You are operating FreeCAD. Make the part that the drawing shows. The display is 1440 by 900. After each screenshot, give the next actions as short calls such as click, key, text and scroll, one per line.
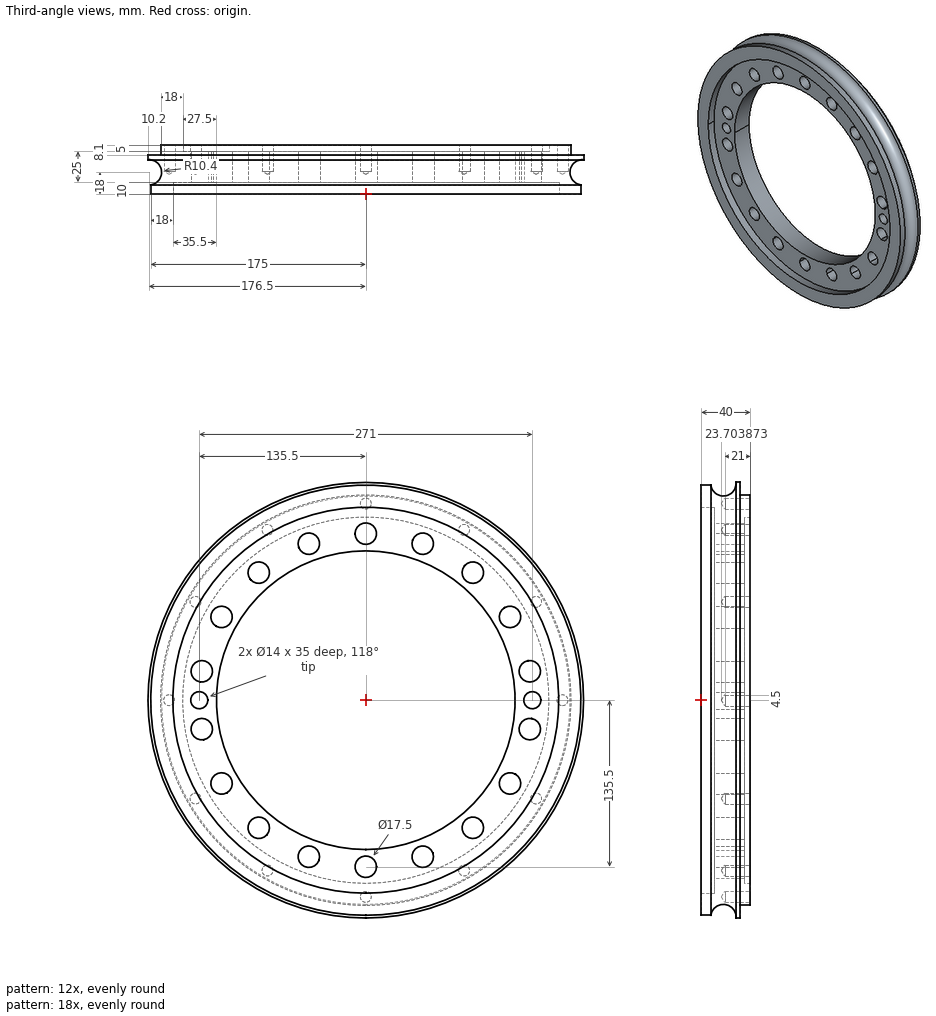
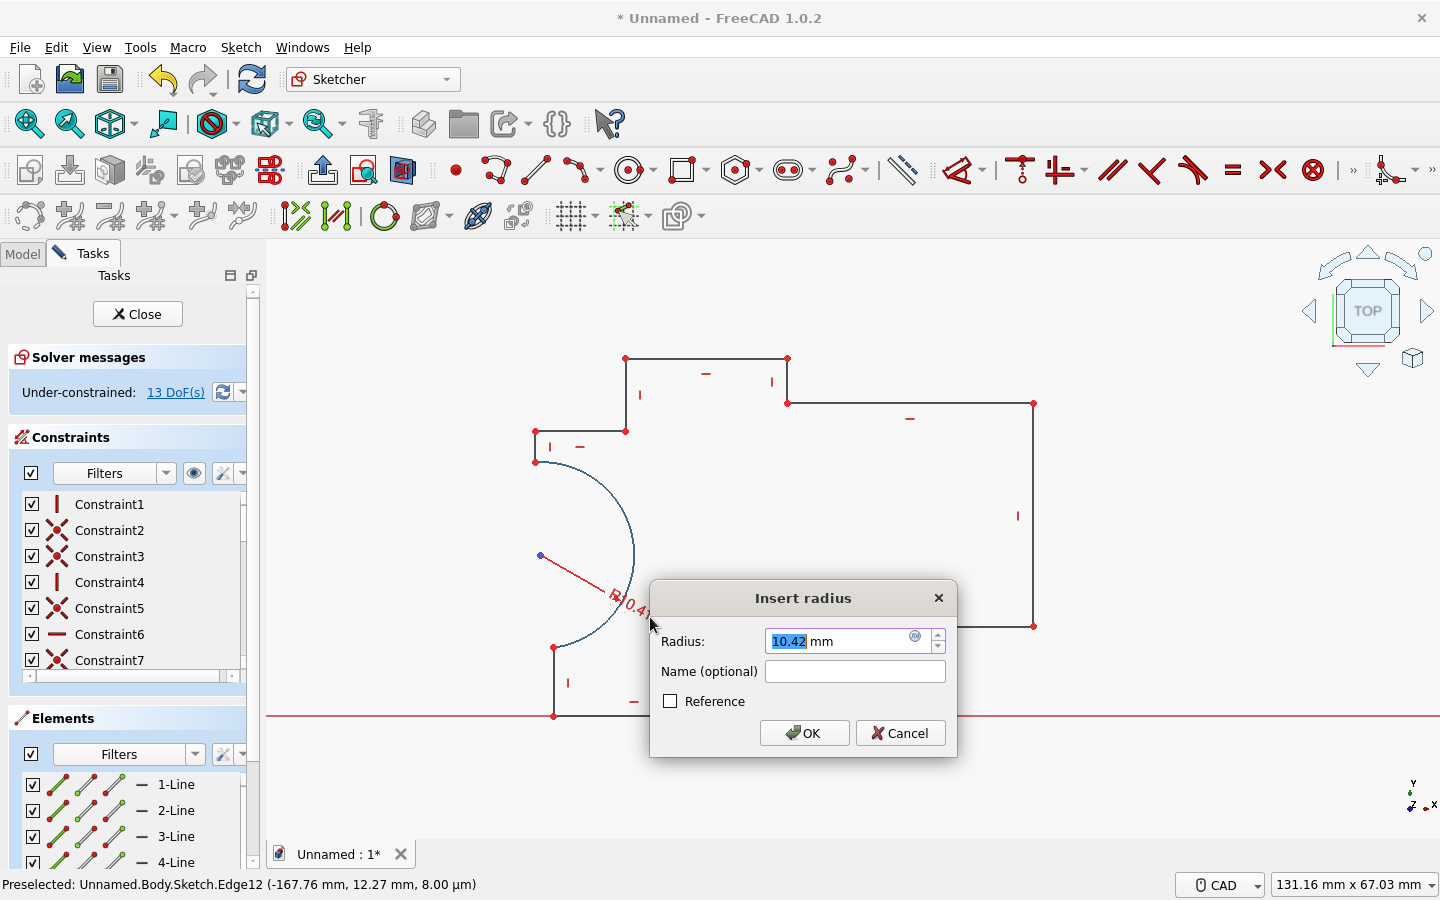
text(10.4)
key(Return)
key(Escape)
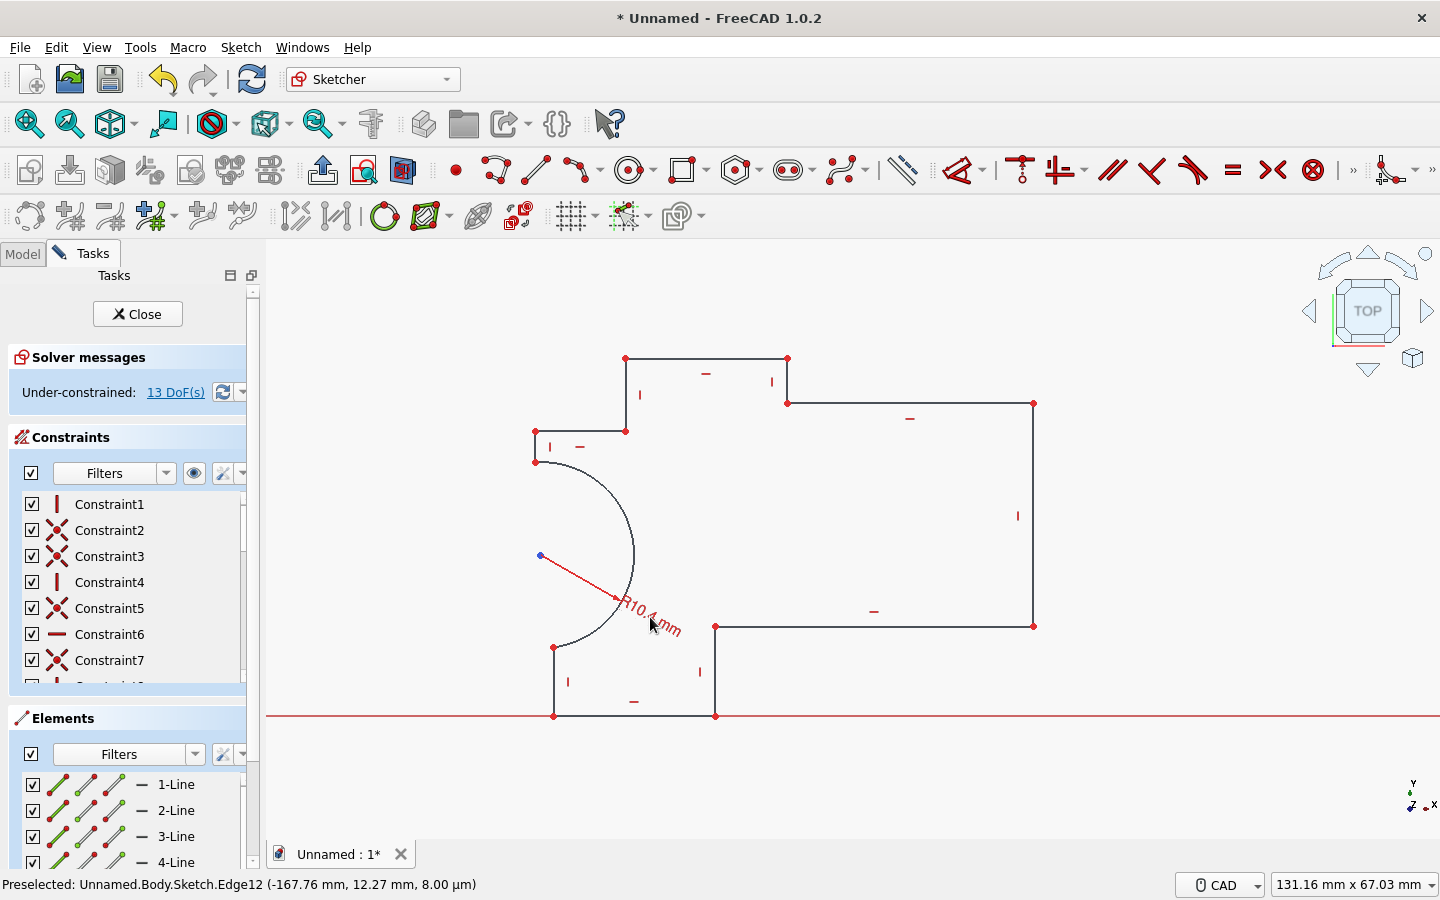
click(554, 716)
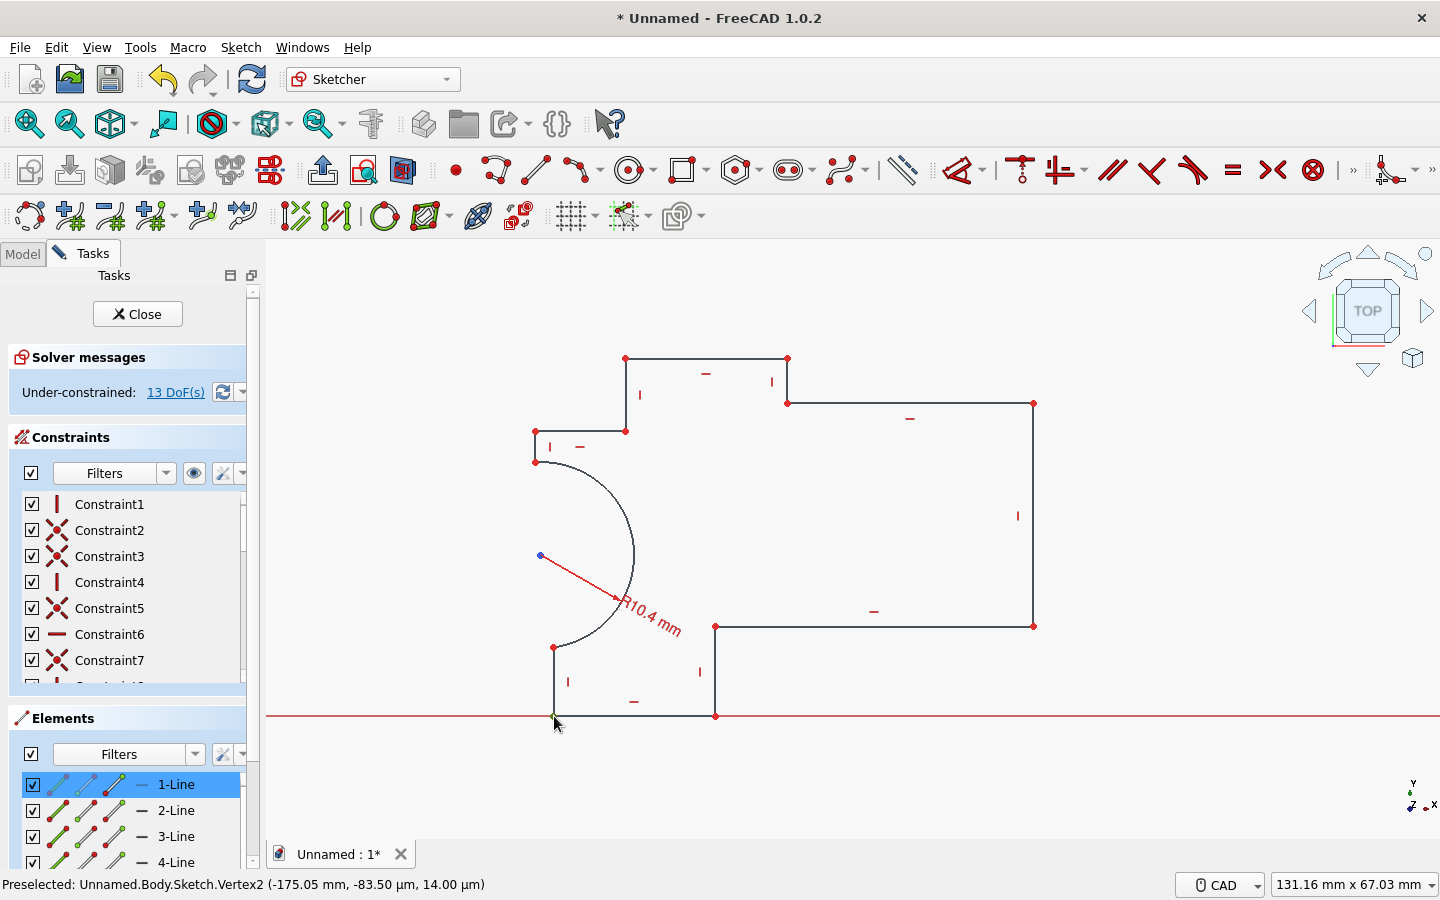
click(364, 716)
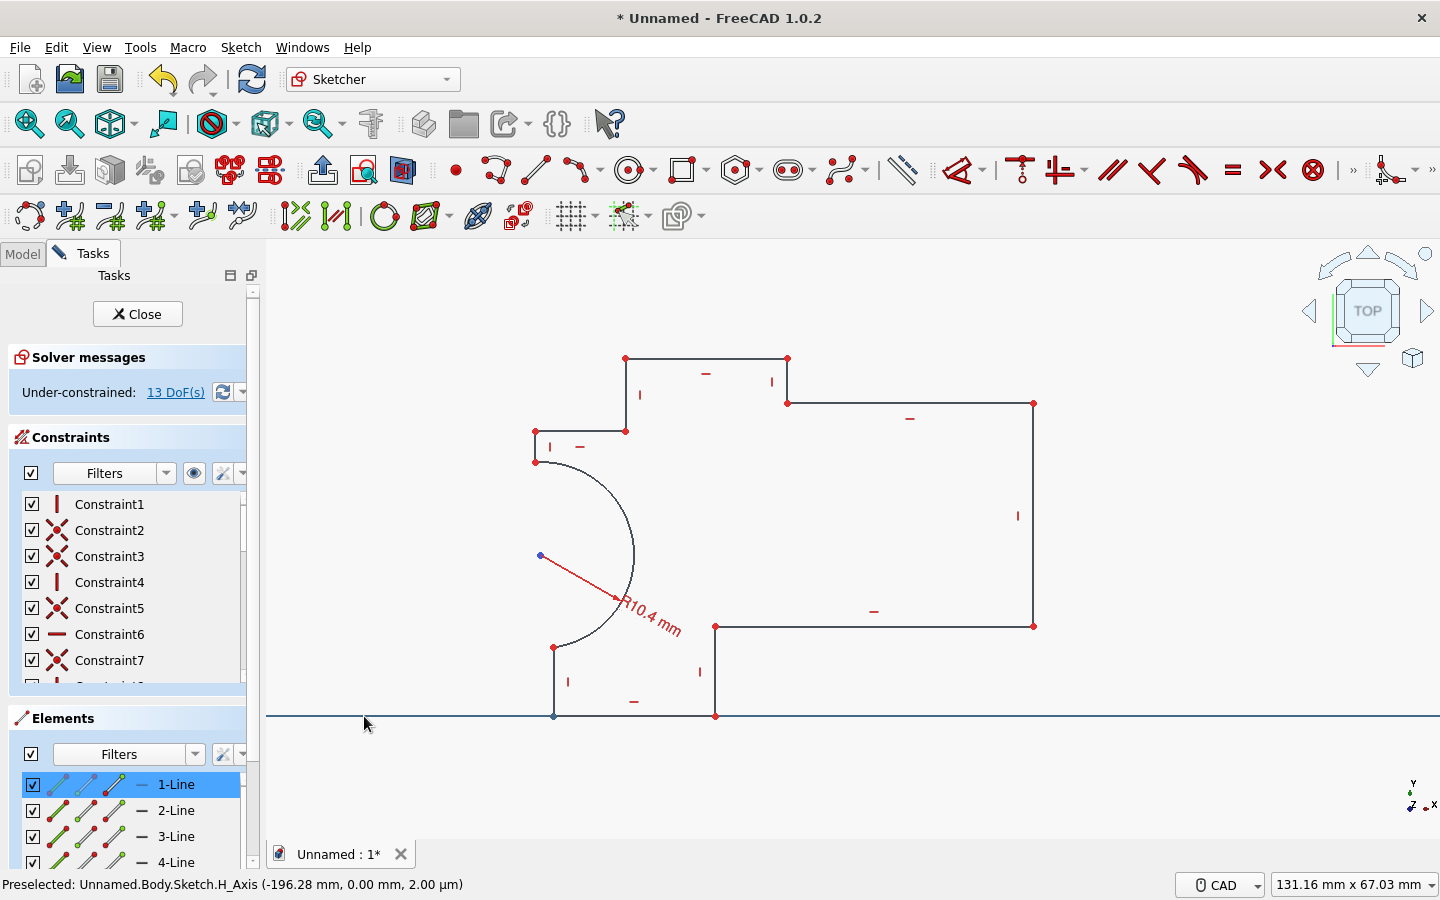
click(1020, 170)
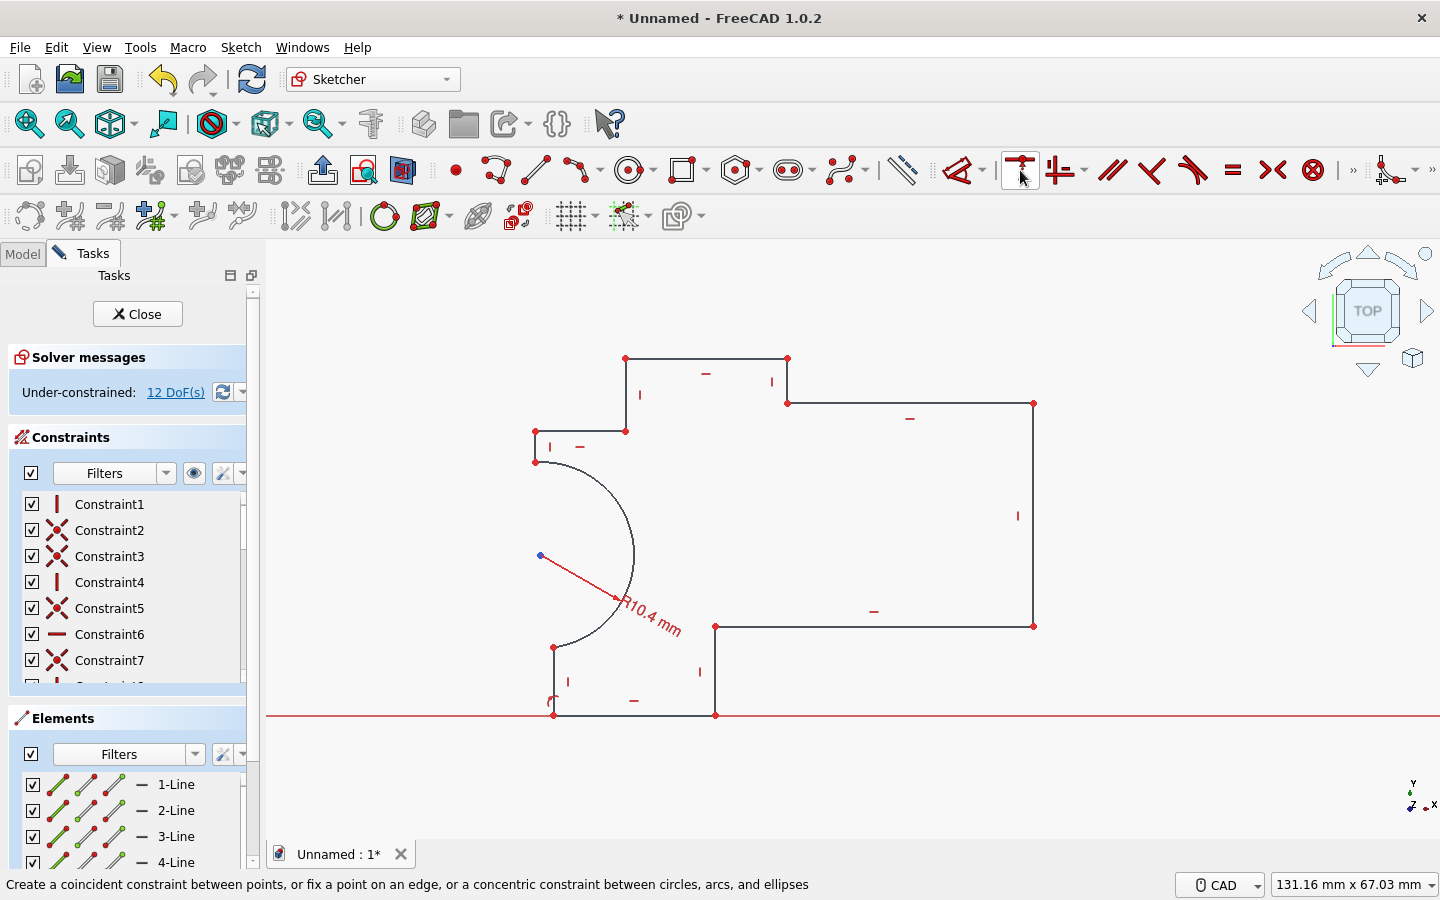
click(958, 170)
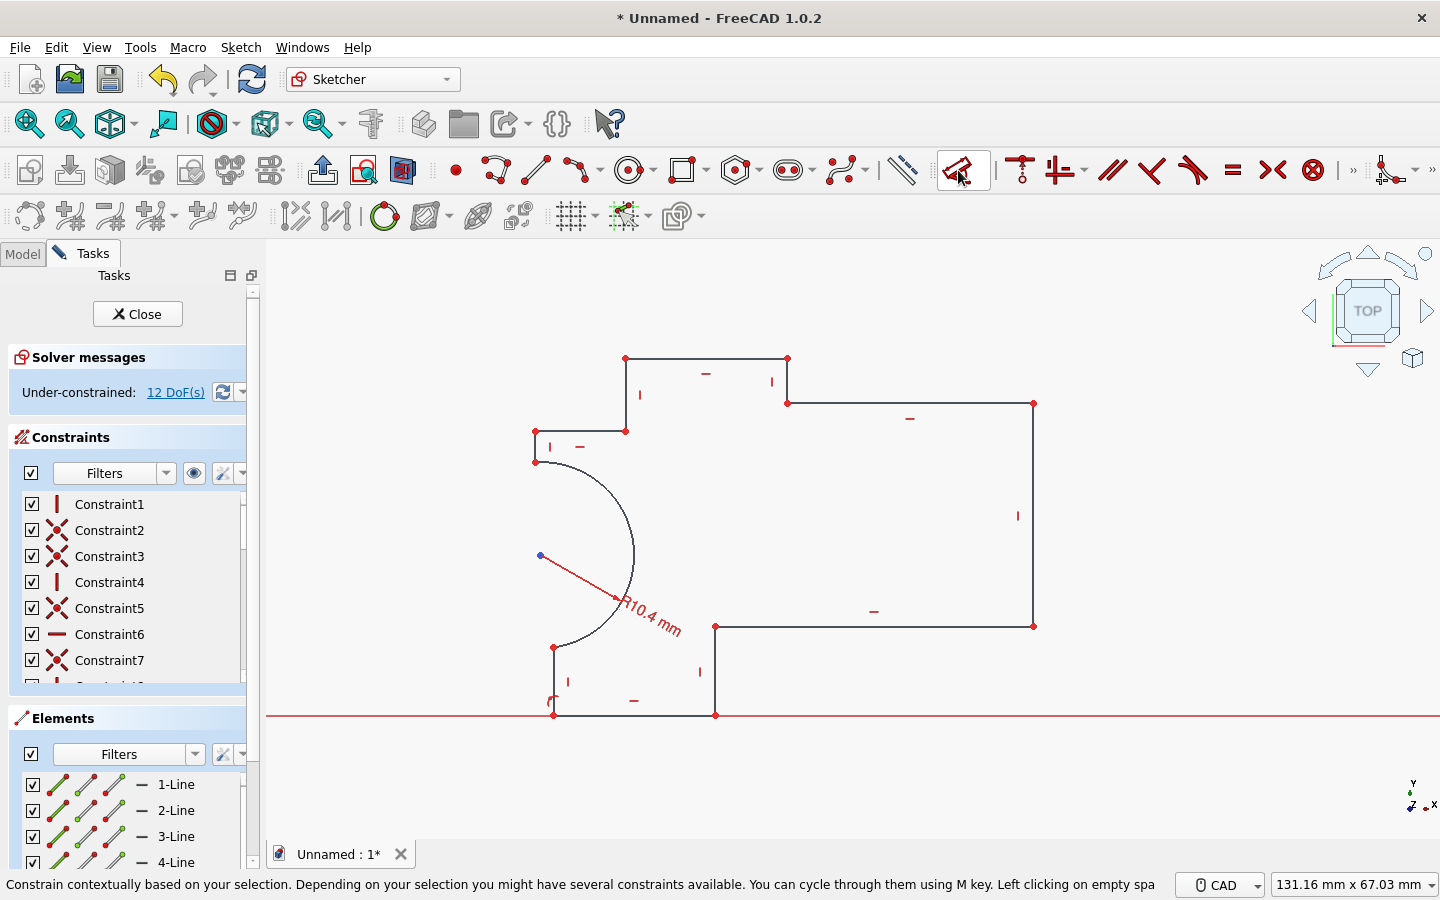
click(787, 390)
click(821, 381)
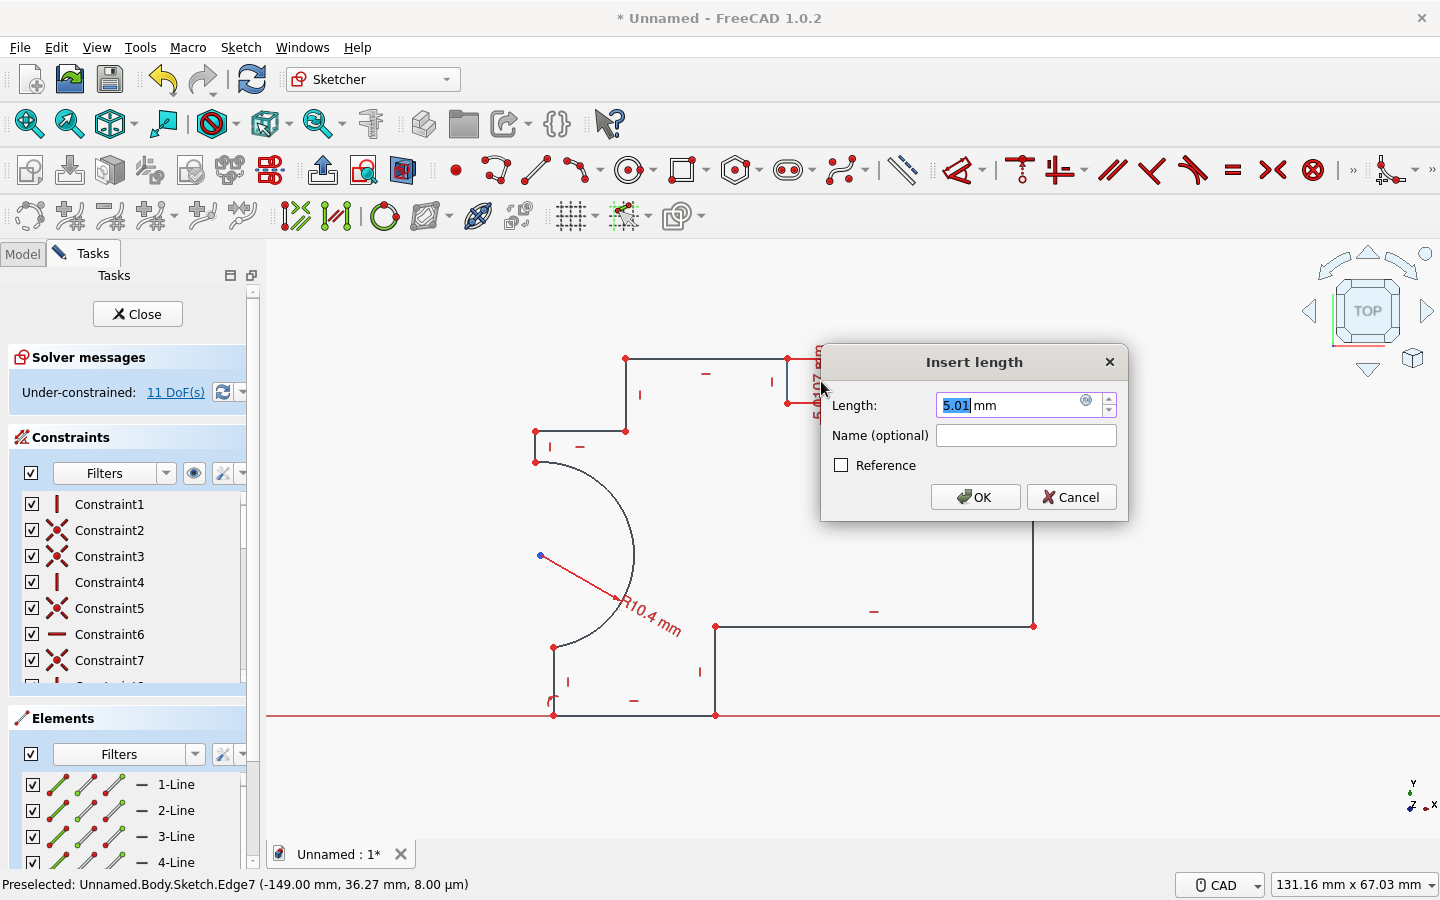
text(5)
key(Return)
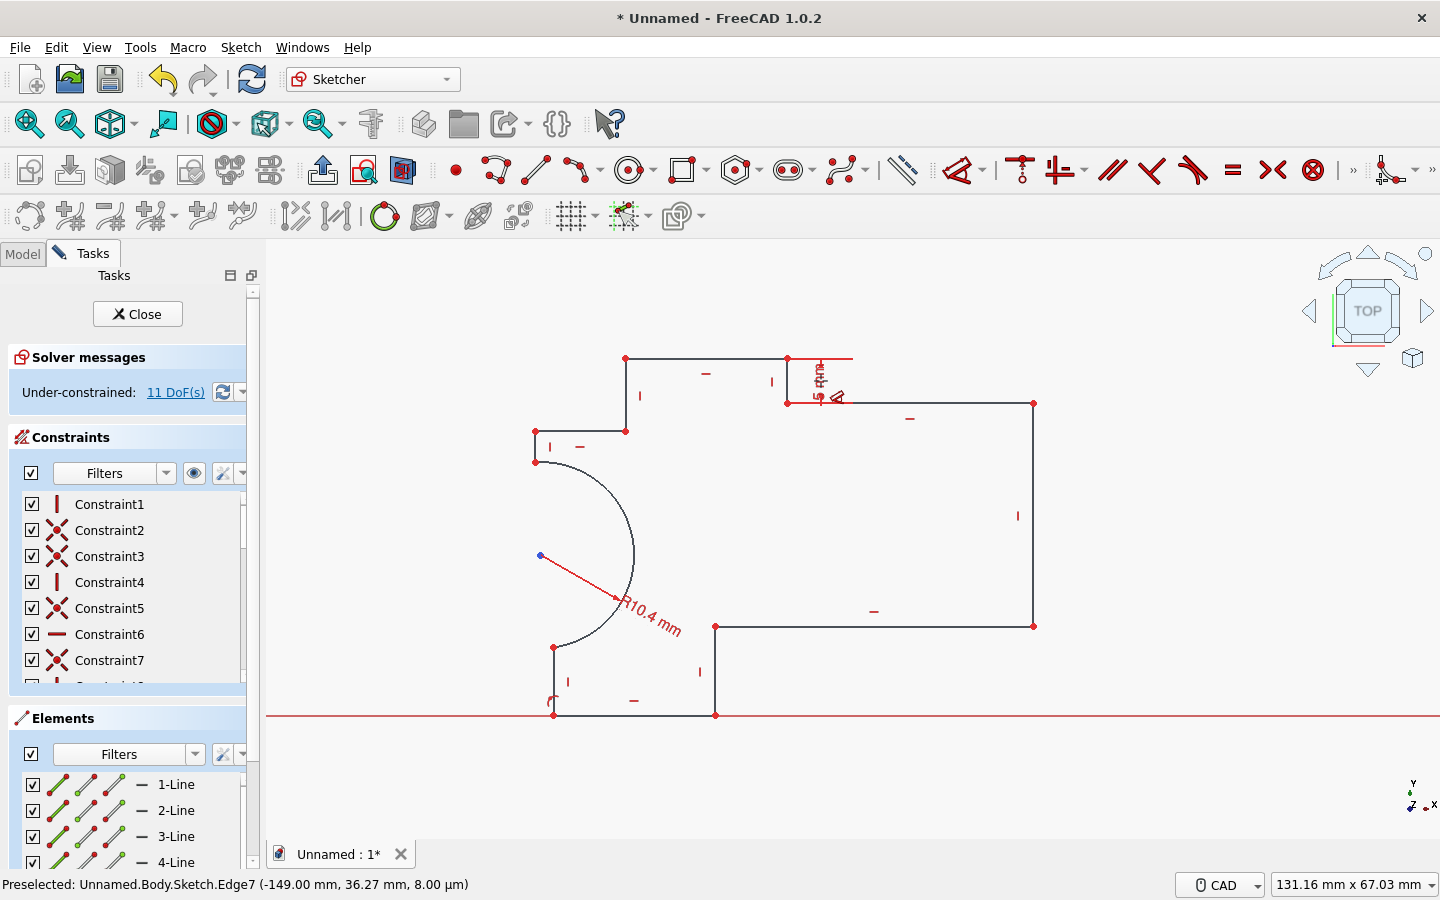
click(602, 716)
click(635, 750)